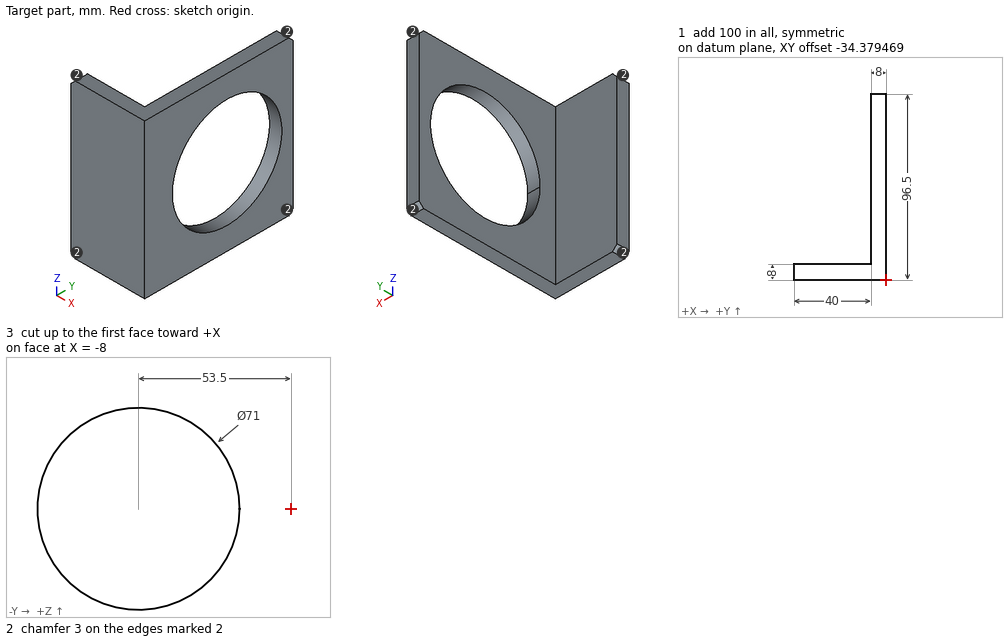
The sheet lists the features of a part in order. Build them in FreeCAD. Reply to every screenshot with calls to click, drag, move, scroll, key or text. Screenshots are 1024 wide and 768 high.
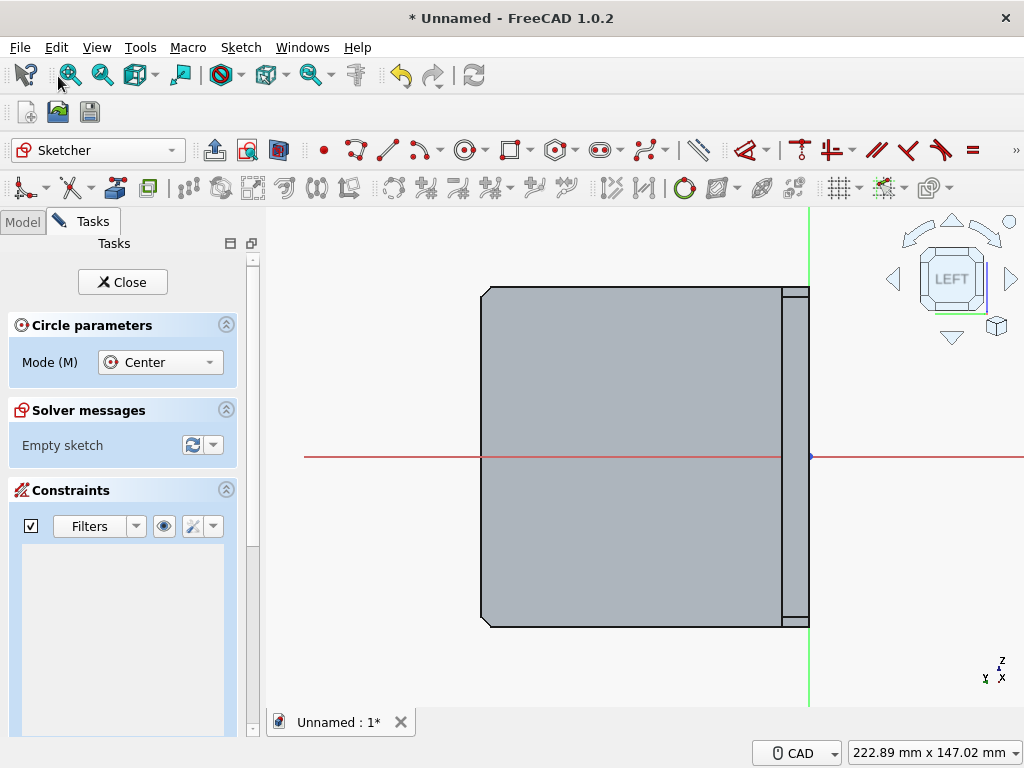
click(627, 457)
move(713, 372)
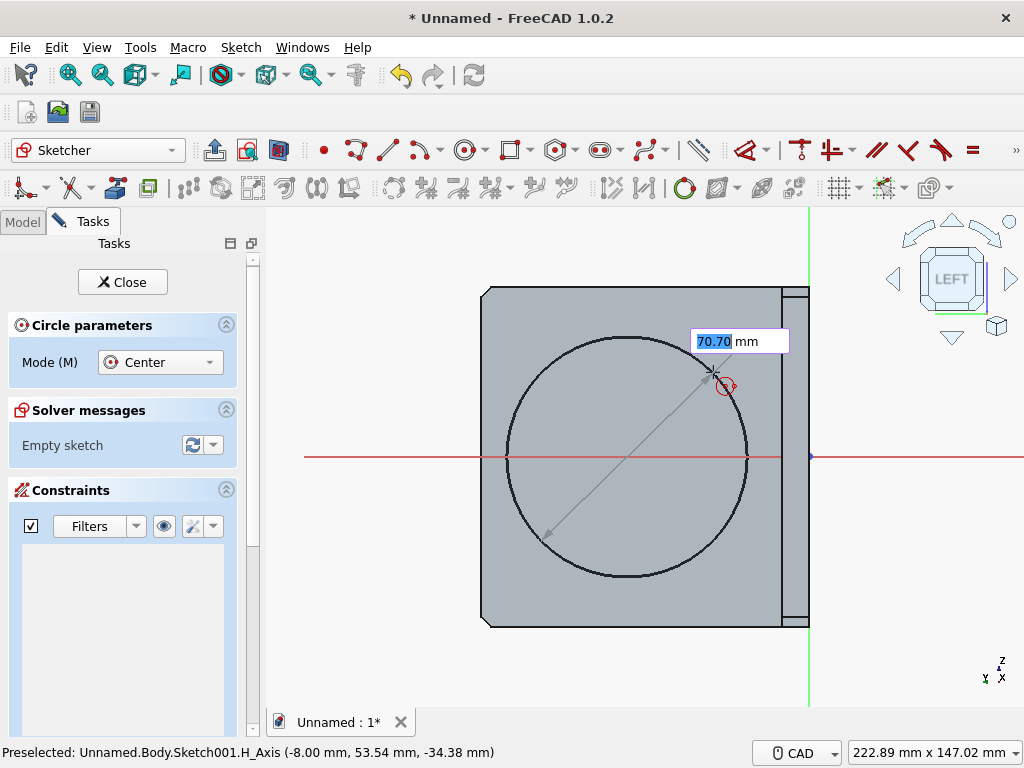
text(71)
key(Return)
key(Escape)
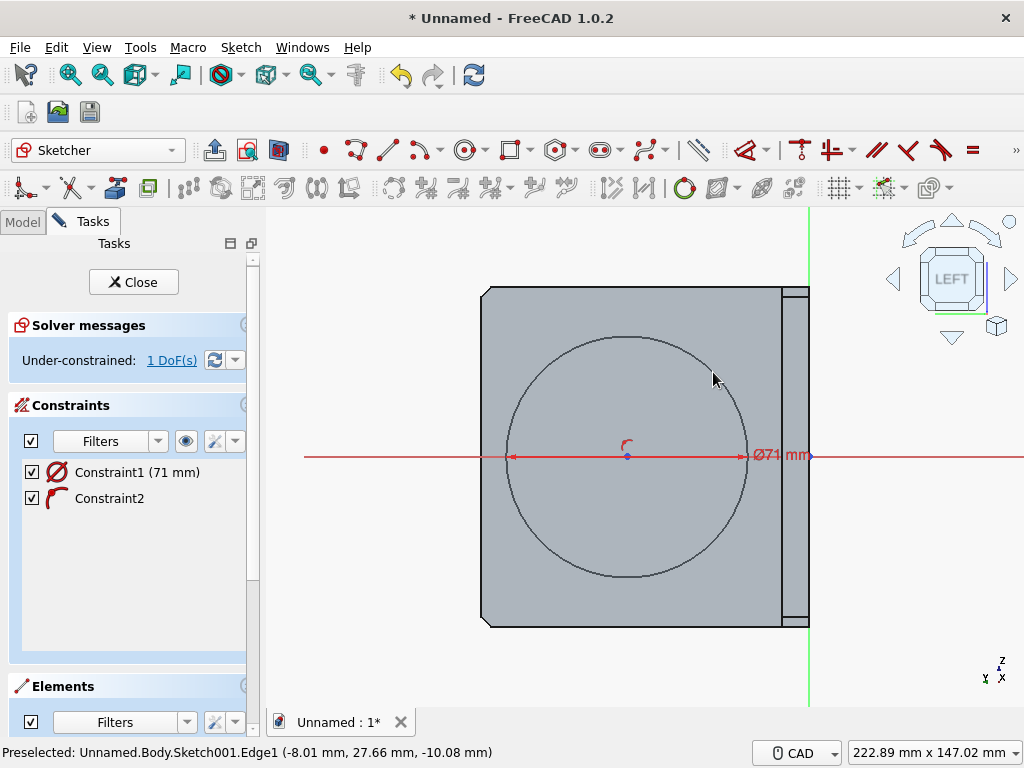
key(d)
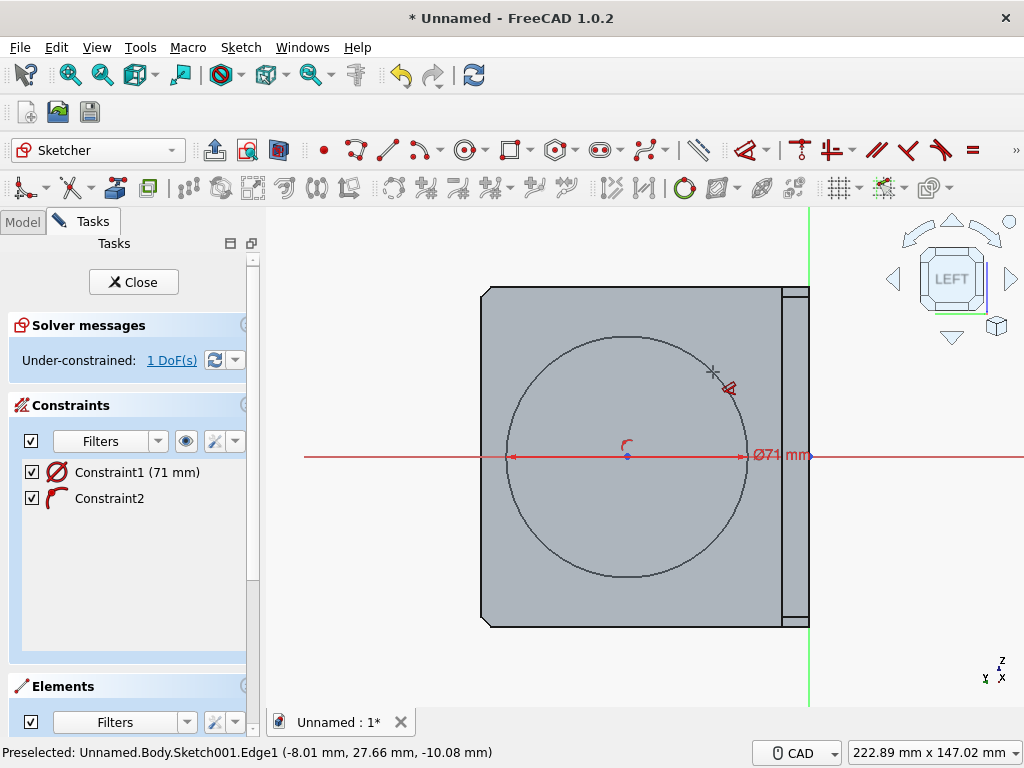
click(627, 457)
click(718, 491)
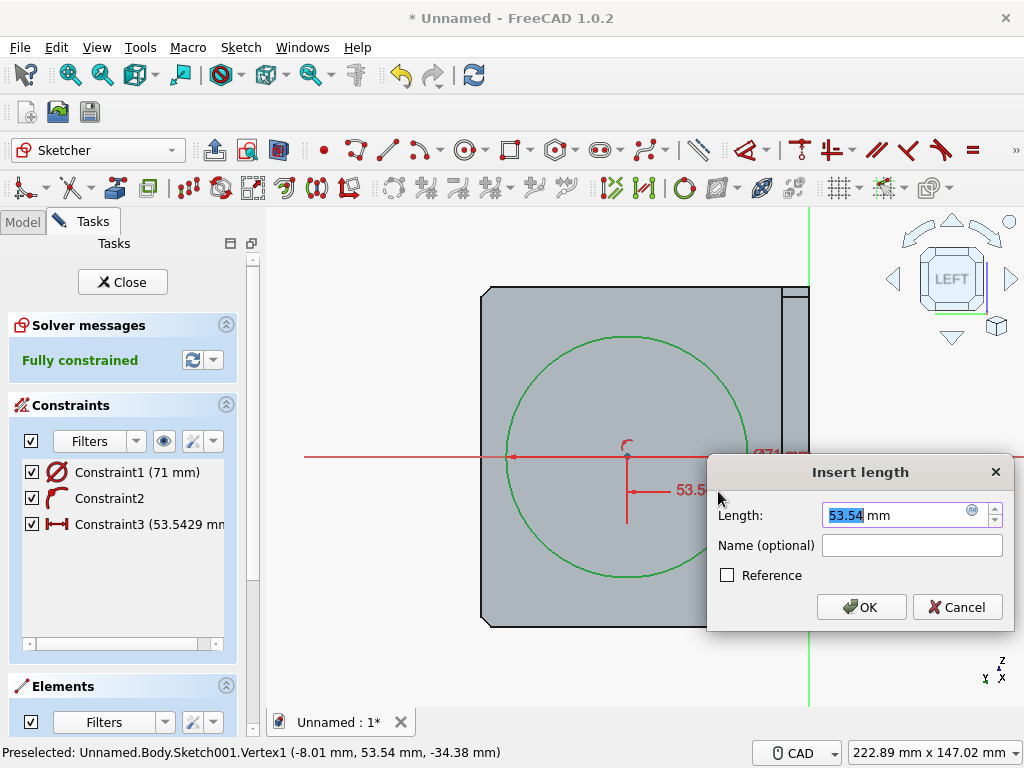
text(53.5)
key(Return)
key(Escape)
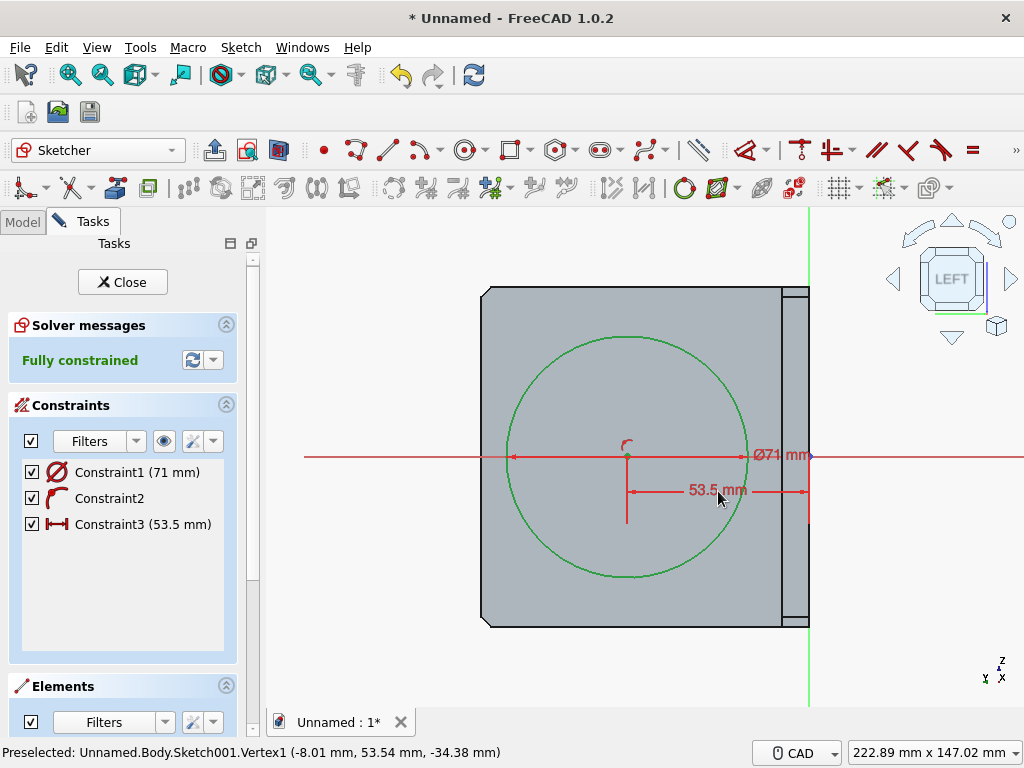
click(123, 282)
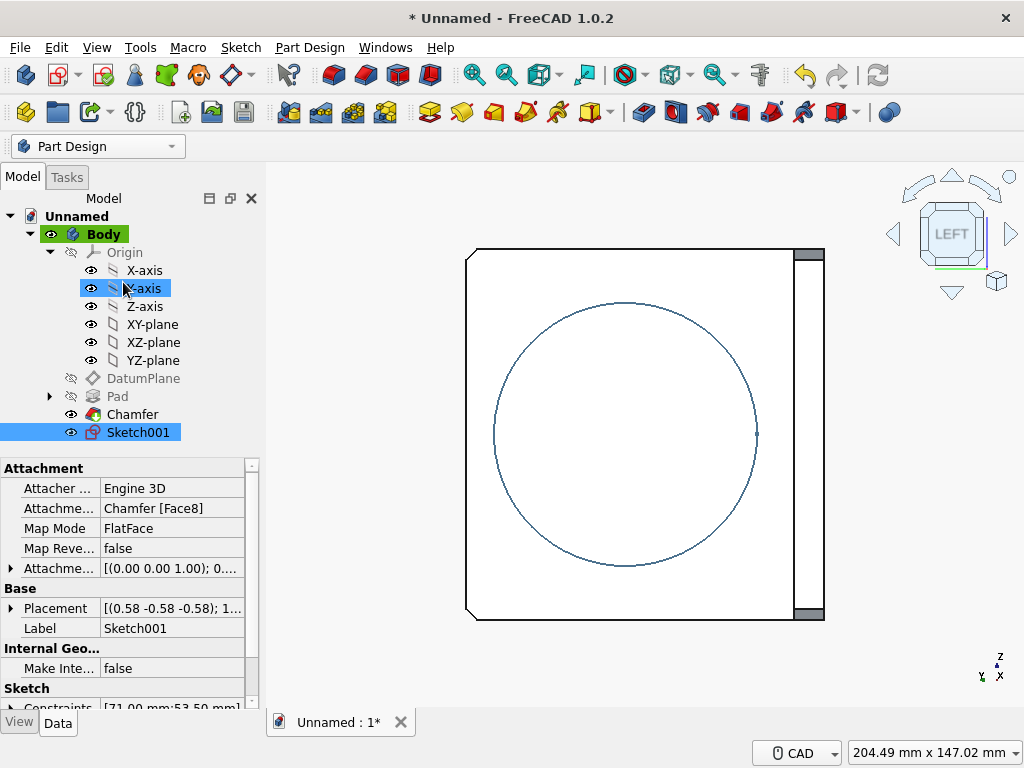
click(644, 112)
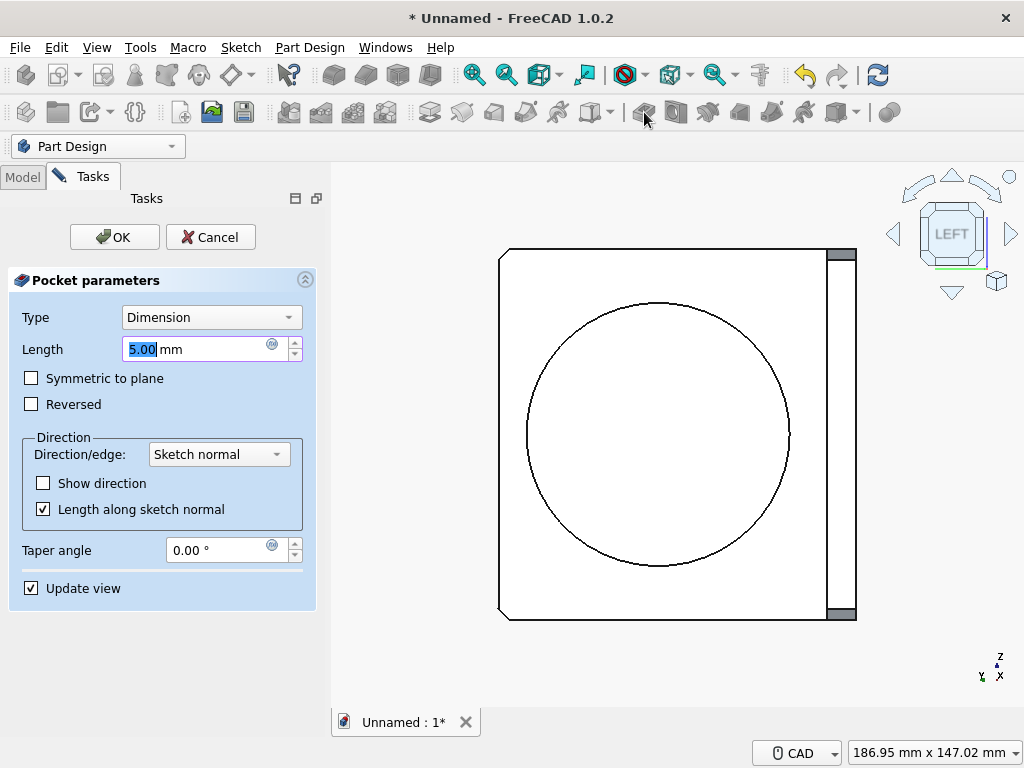
click(212, 318)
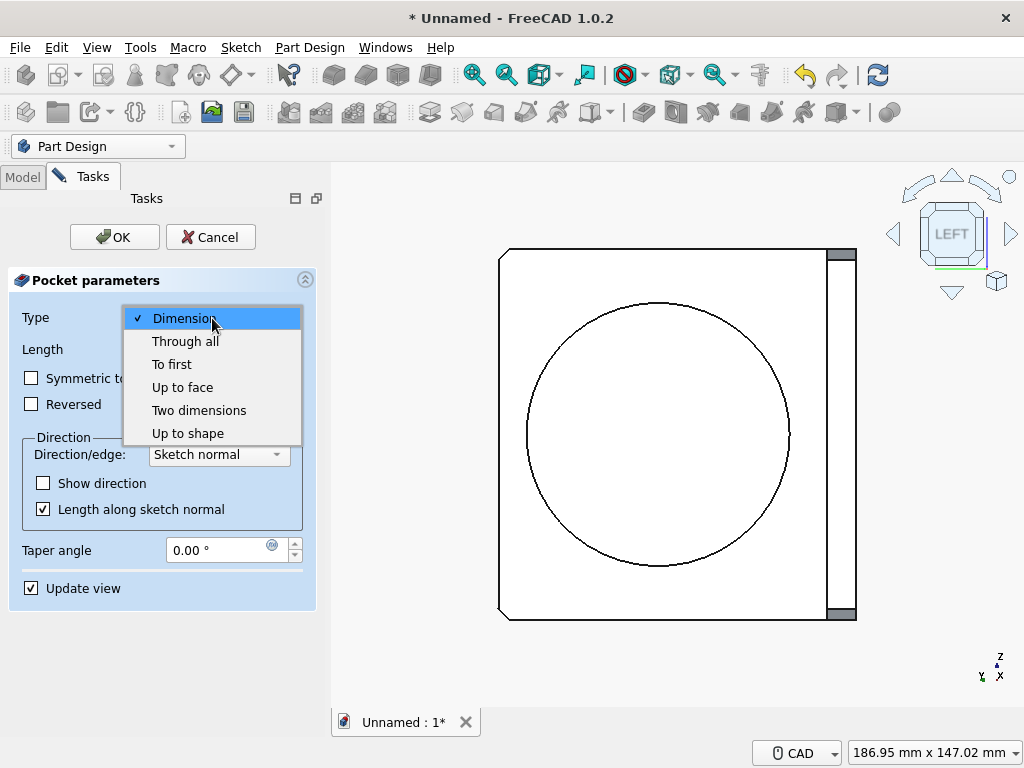
click(212, 364)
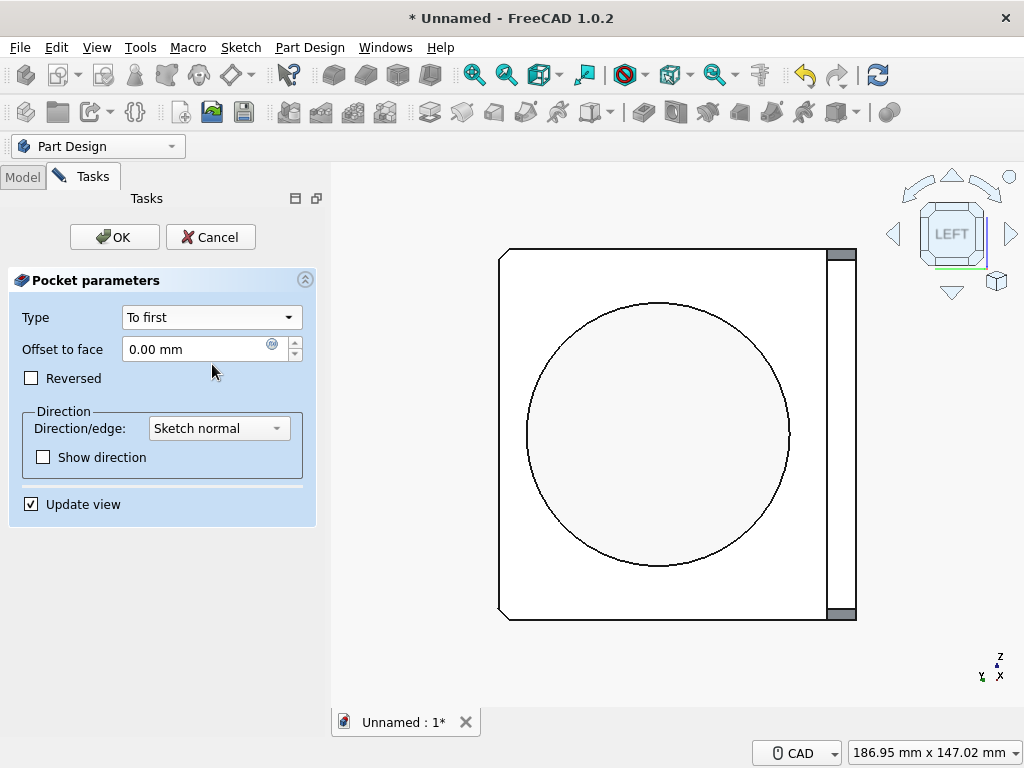
click(115, 237)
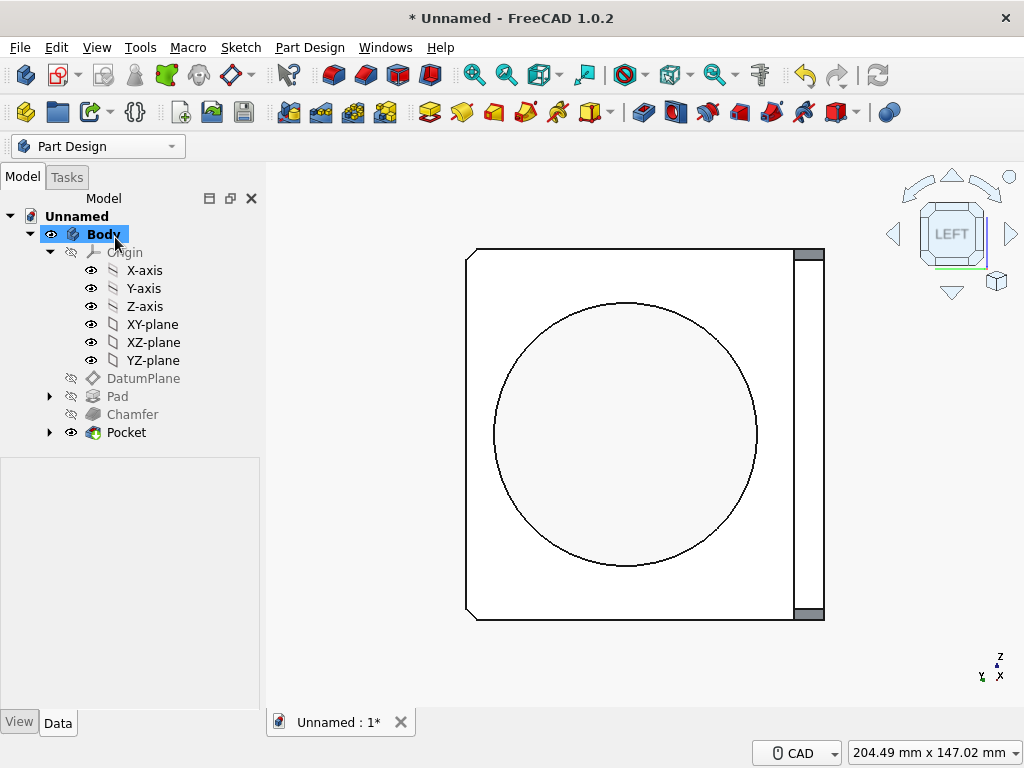
key(0)